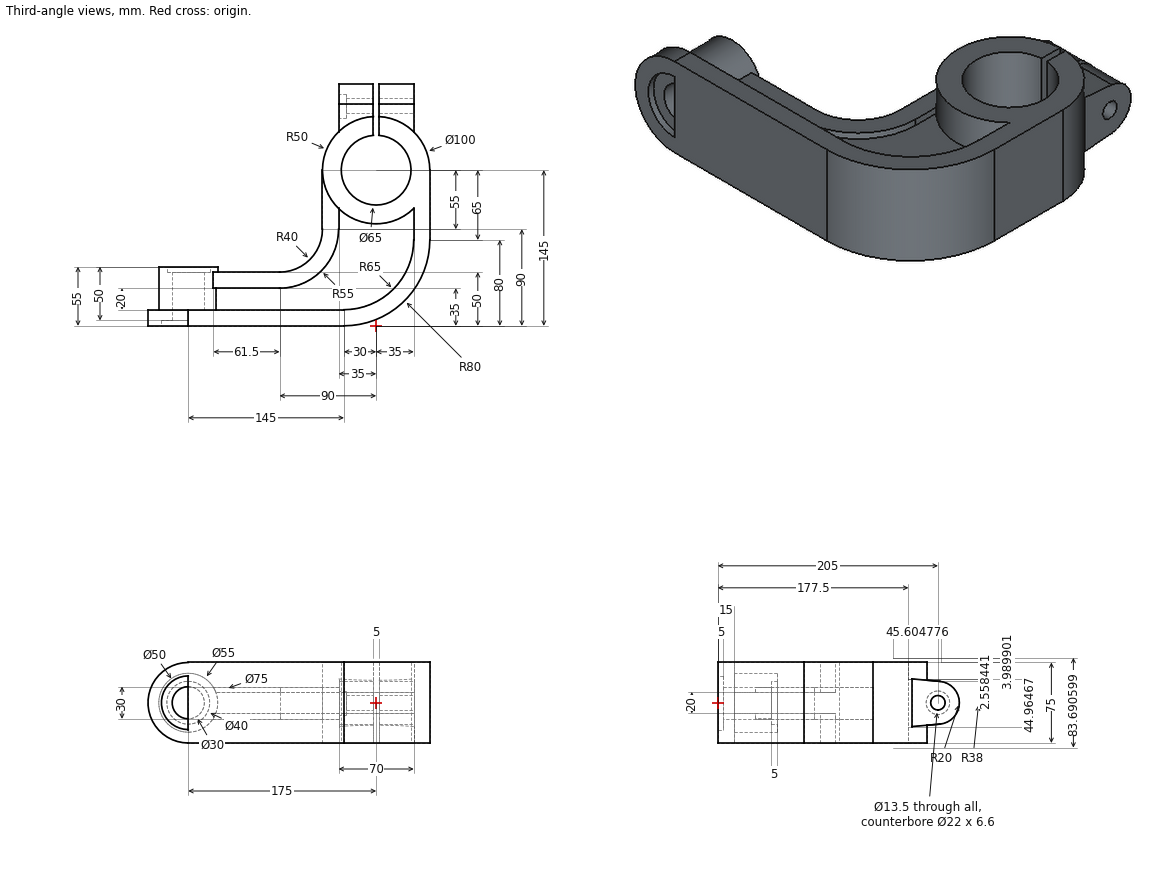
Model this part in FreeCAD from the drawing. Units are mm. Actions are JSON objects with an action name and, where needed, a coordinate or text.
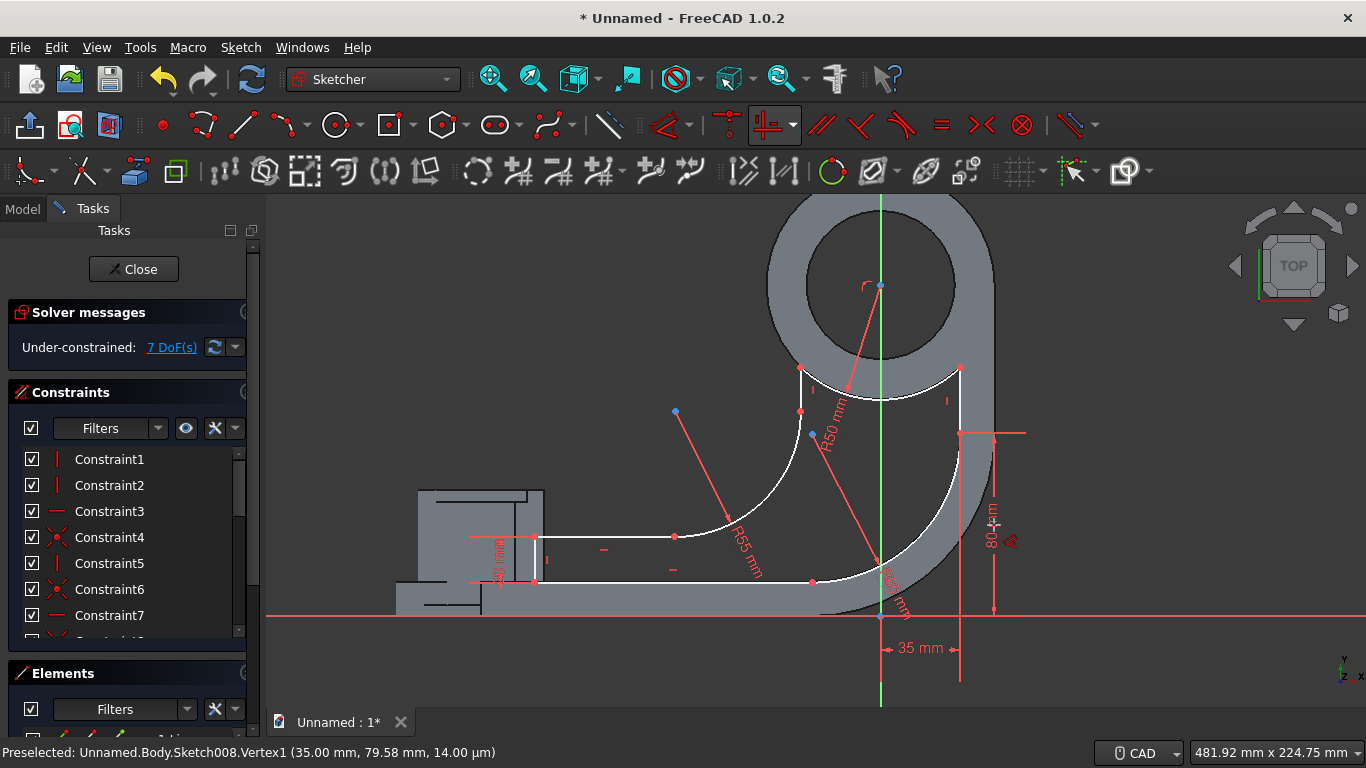
{"action": "left_click", "coordinate": [801, 367]}
{"action": "left_click", "coordinate": [841, 650]}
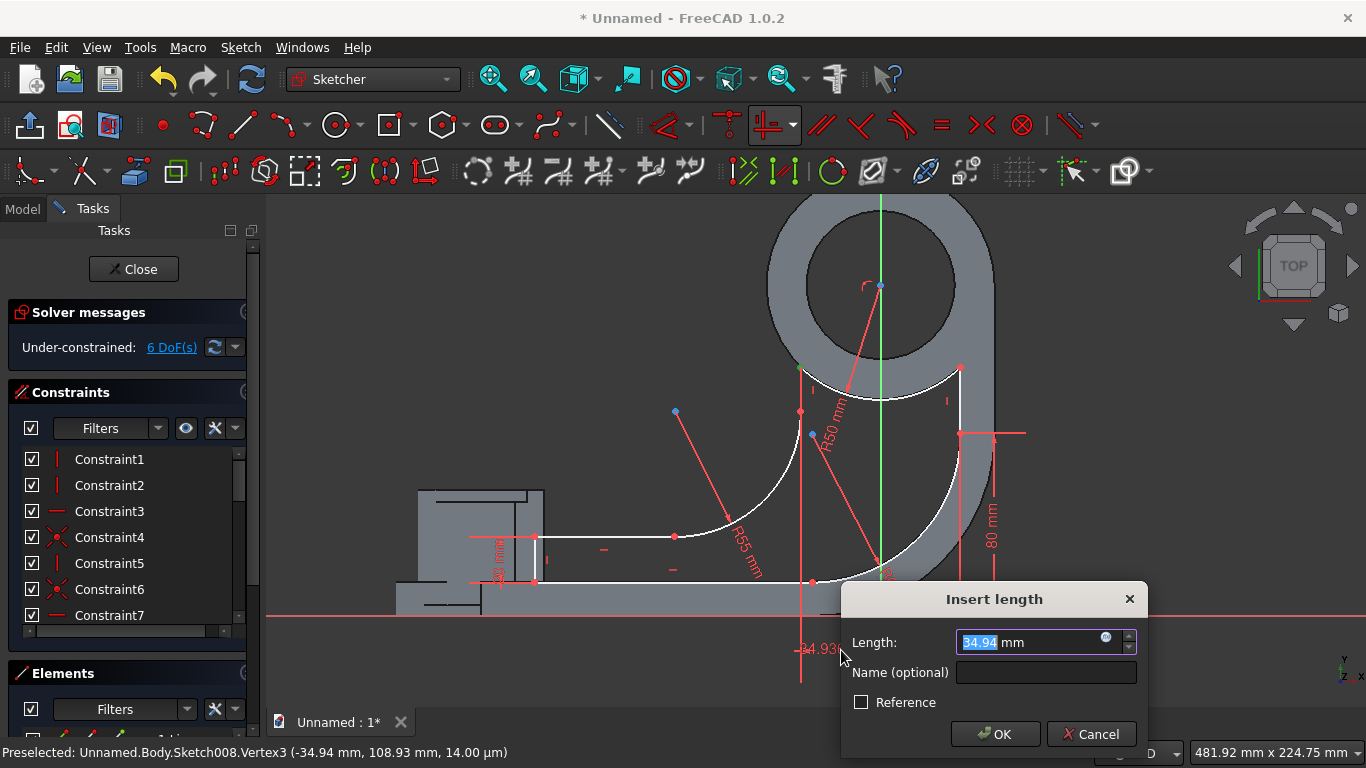
{"action": "type", "text": "35"}
{"action": "key", "text": "Return"}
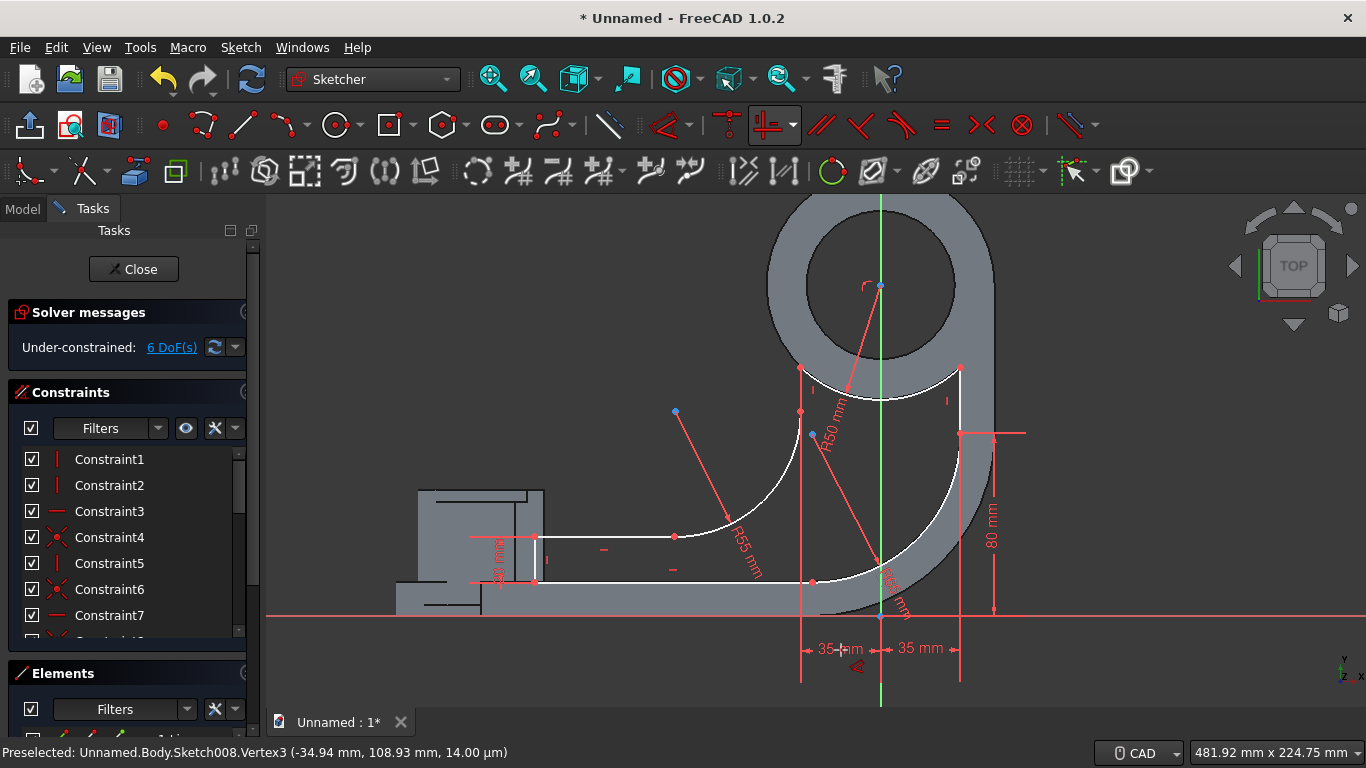
{"action": "left_click", "coordinate": [801, 411]}
{"action": "left_click", "coordinate": [915, 514]}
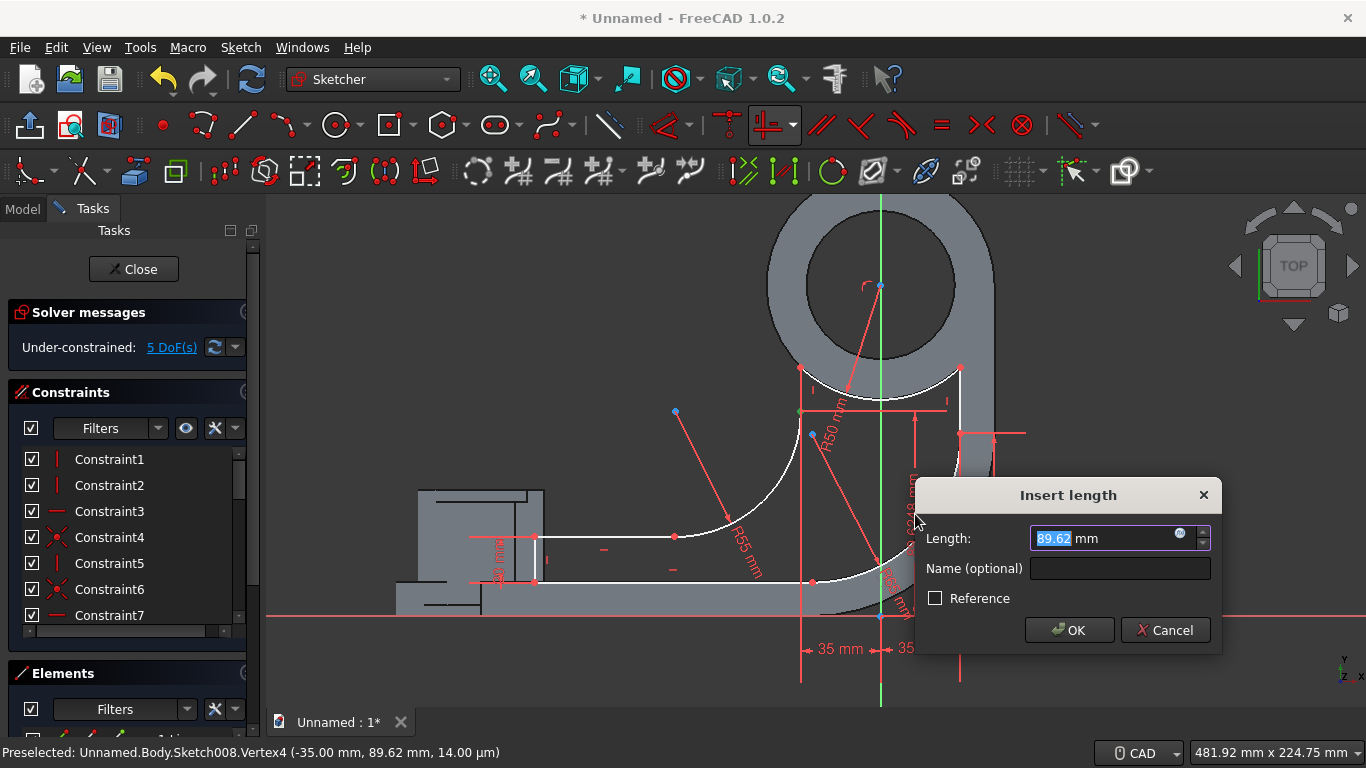
{"action": "type", "text": "90"}
{"action": "key", "text": "Return"}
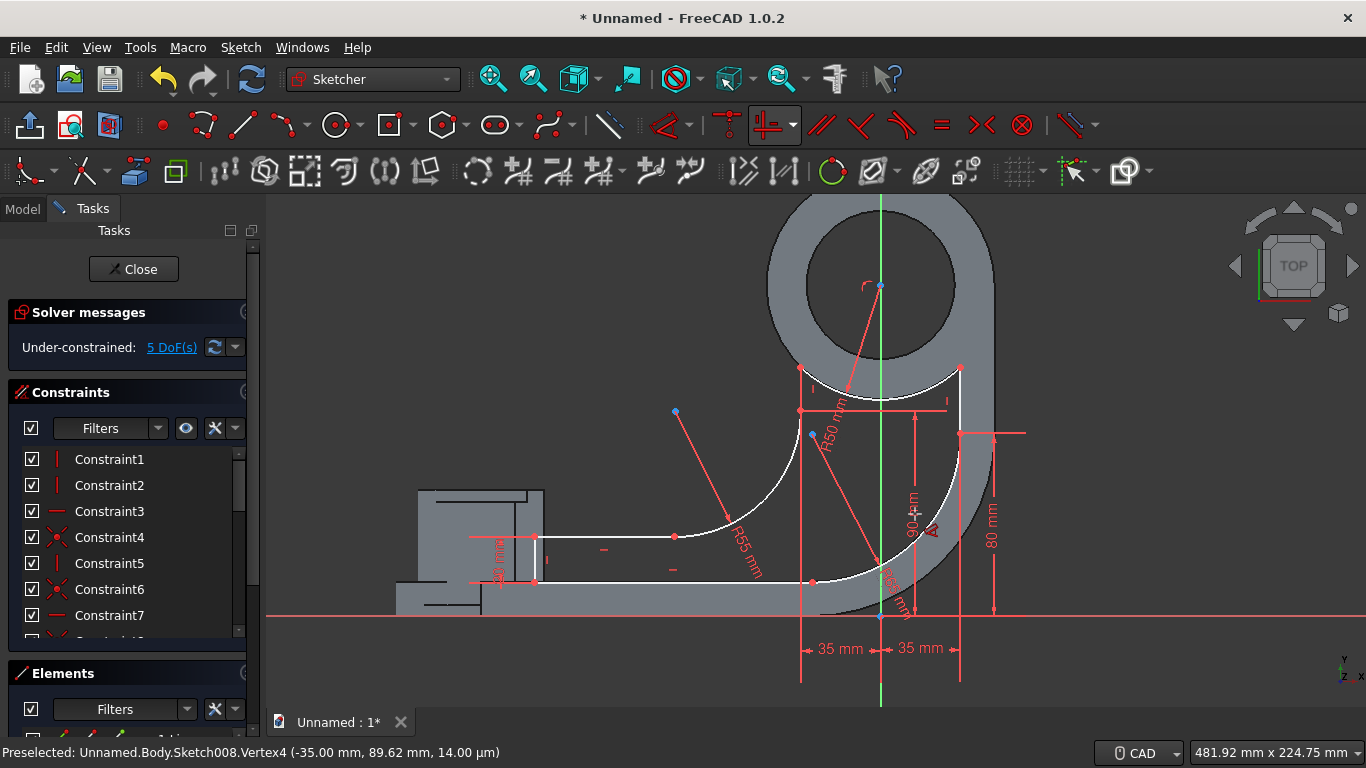
{"action": "left_click", "coordinate": [675, 537]}
{"action": "left_click", "coordinate": [730, 650]}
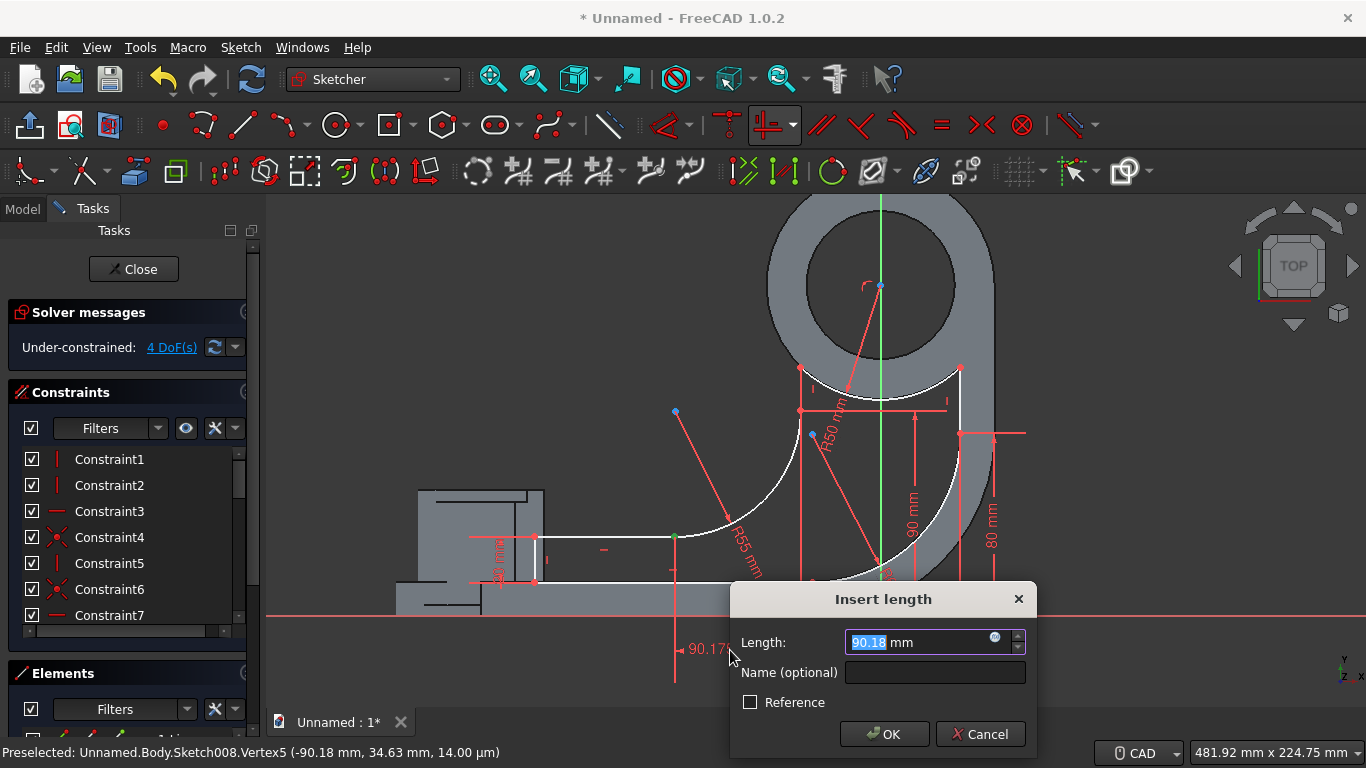
{"action": "type", "text": "90"}
{"action": "key", "text": "Return"}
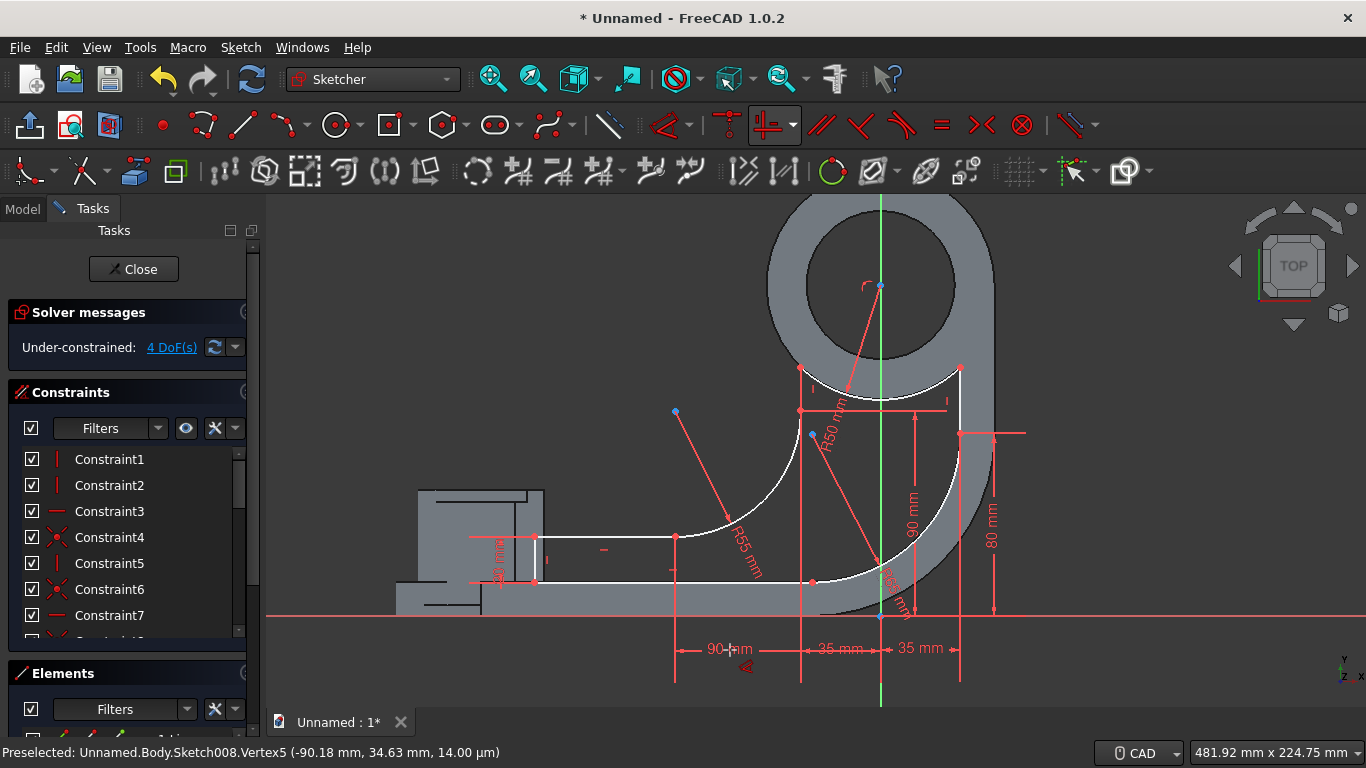
{"action": "left_click", "coordinate": [675, 537]}
{"action": "left_click", "coordinate": [641, 558]}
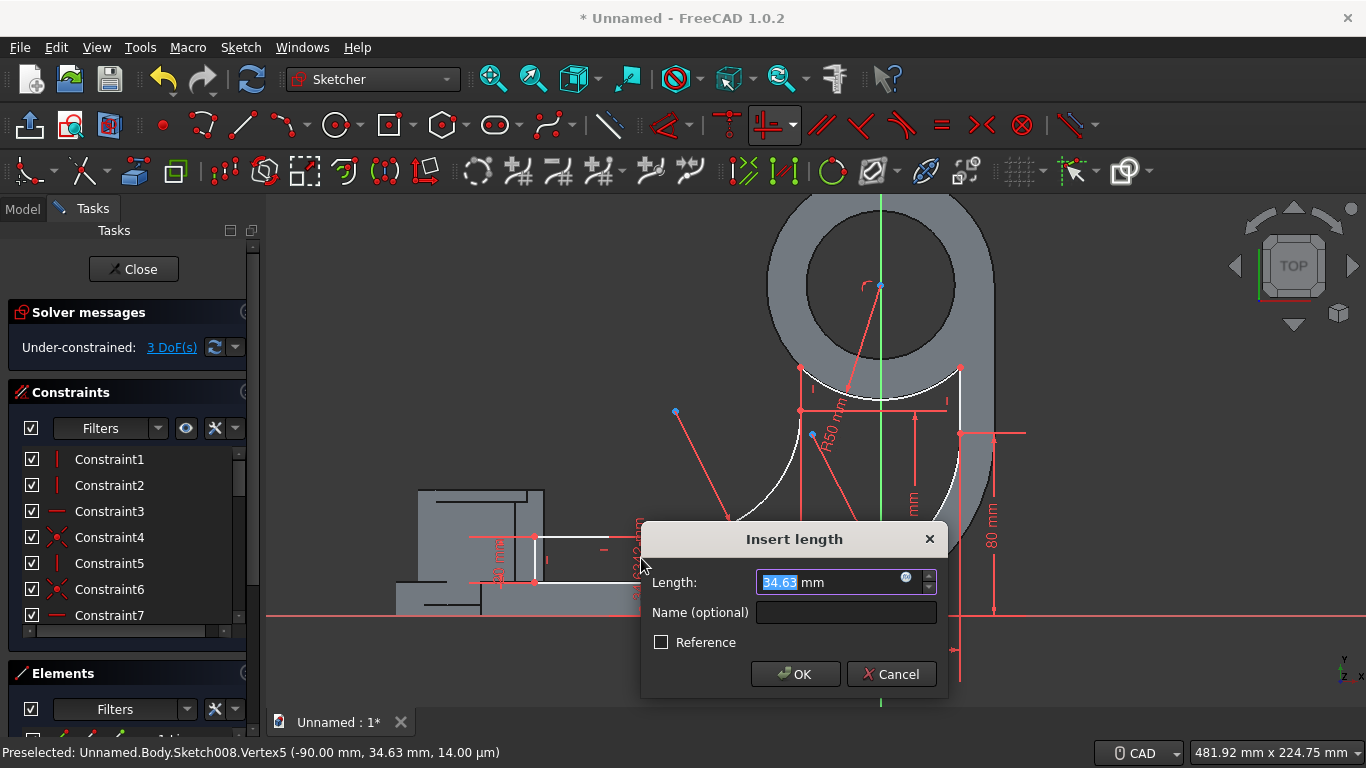
{"action": "type", "text": "35"}
{"action": "key", "text": "Return"}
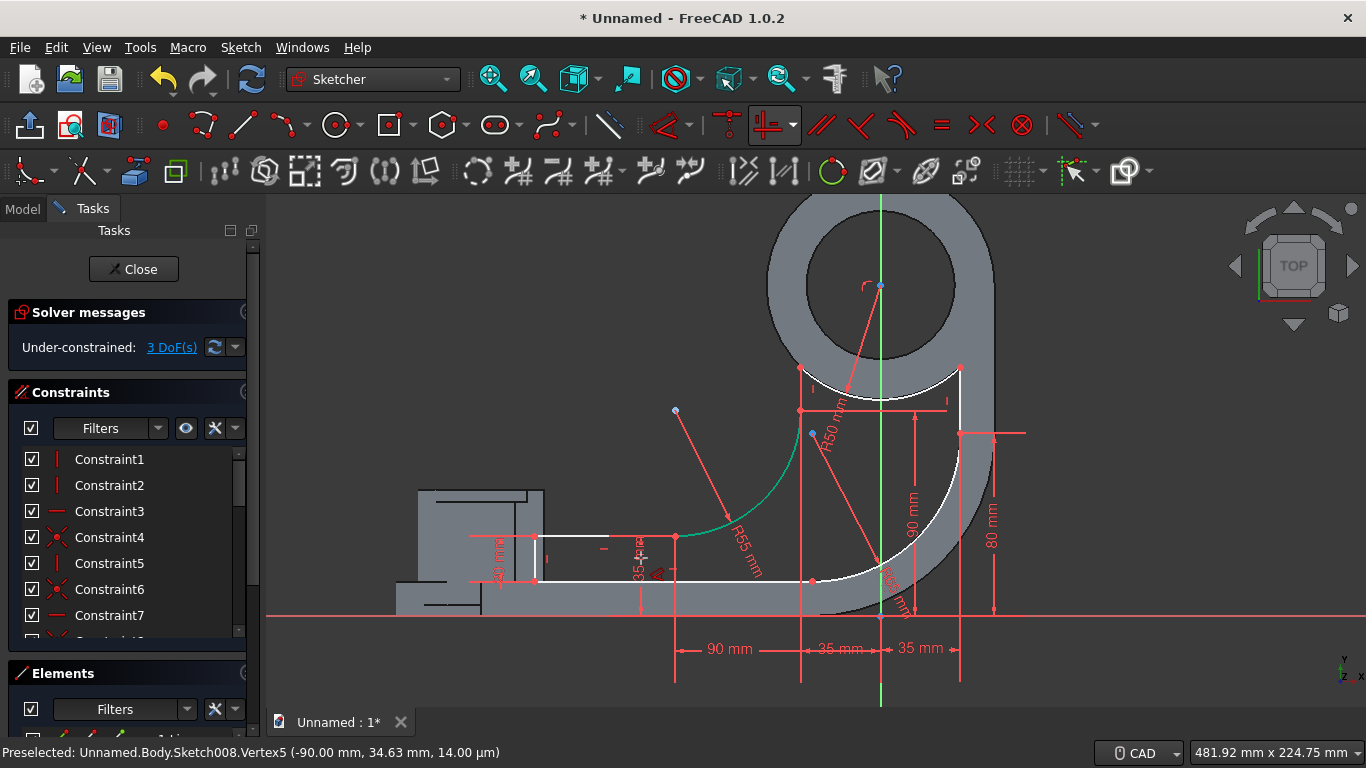
{"action": "left_click", "coordinate": [812, 582]}
{"action": "left_click", "coordinate": [846, 548]}